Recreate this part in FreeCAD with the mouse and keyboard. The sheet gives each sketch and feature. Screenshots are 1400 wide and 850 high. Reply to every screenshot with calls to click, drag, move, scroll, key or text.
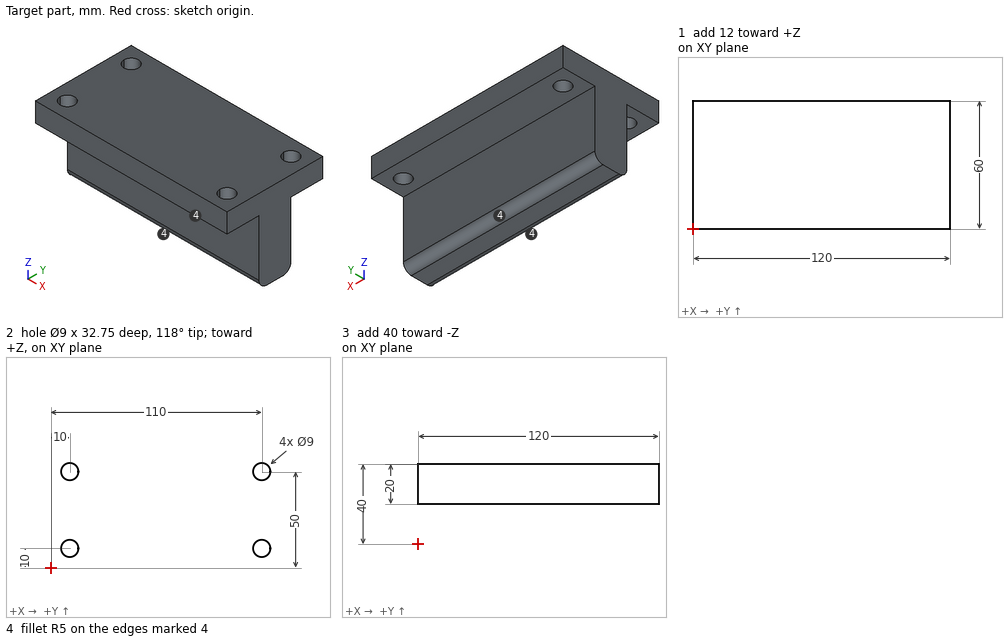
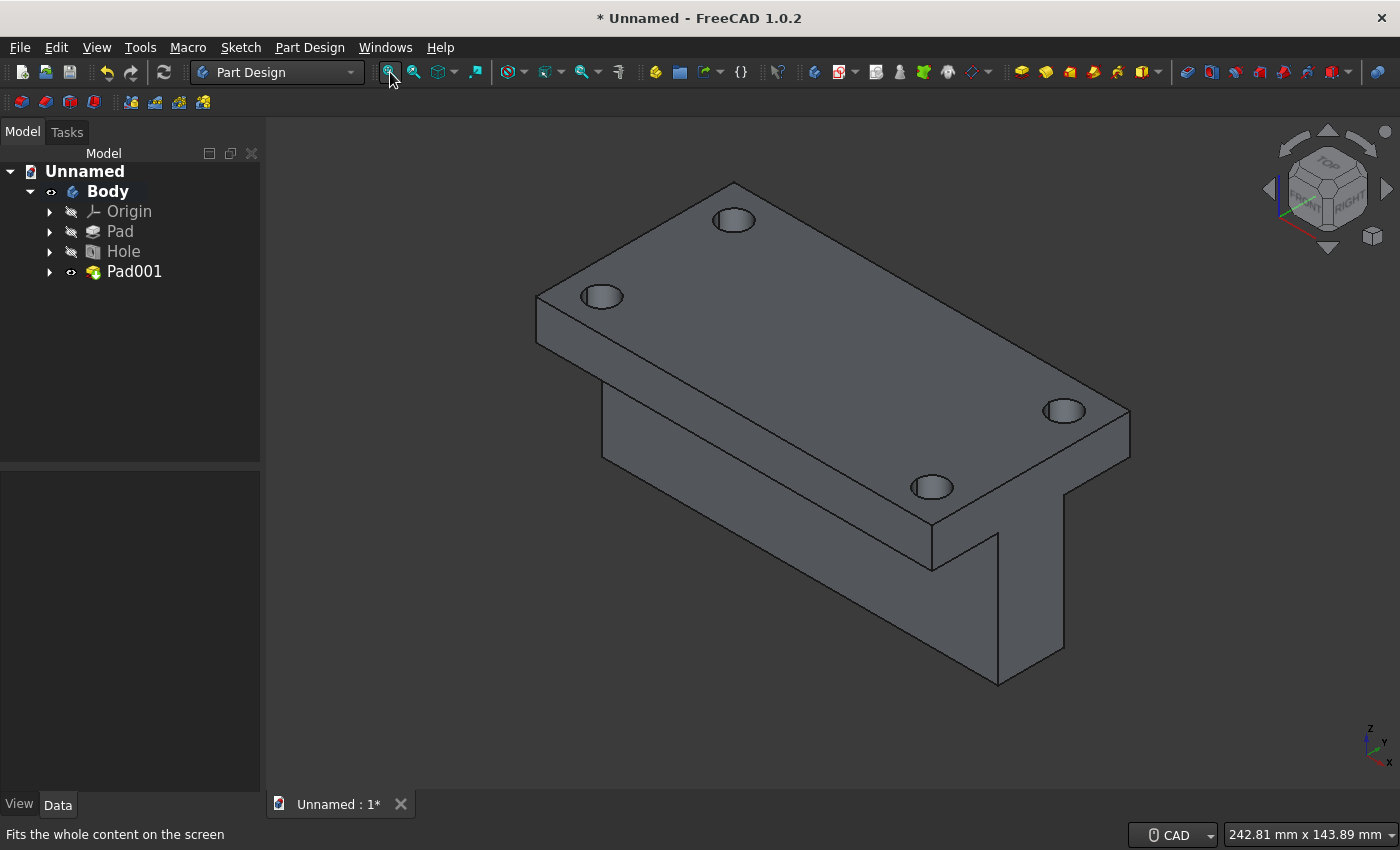
key(2)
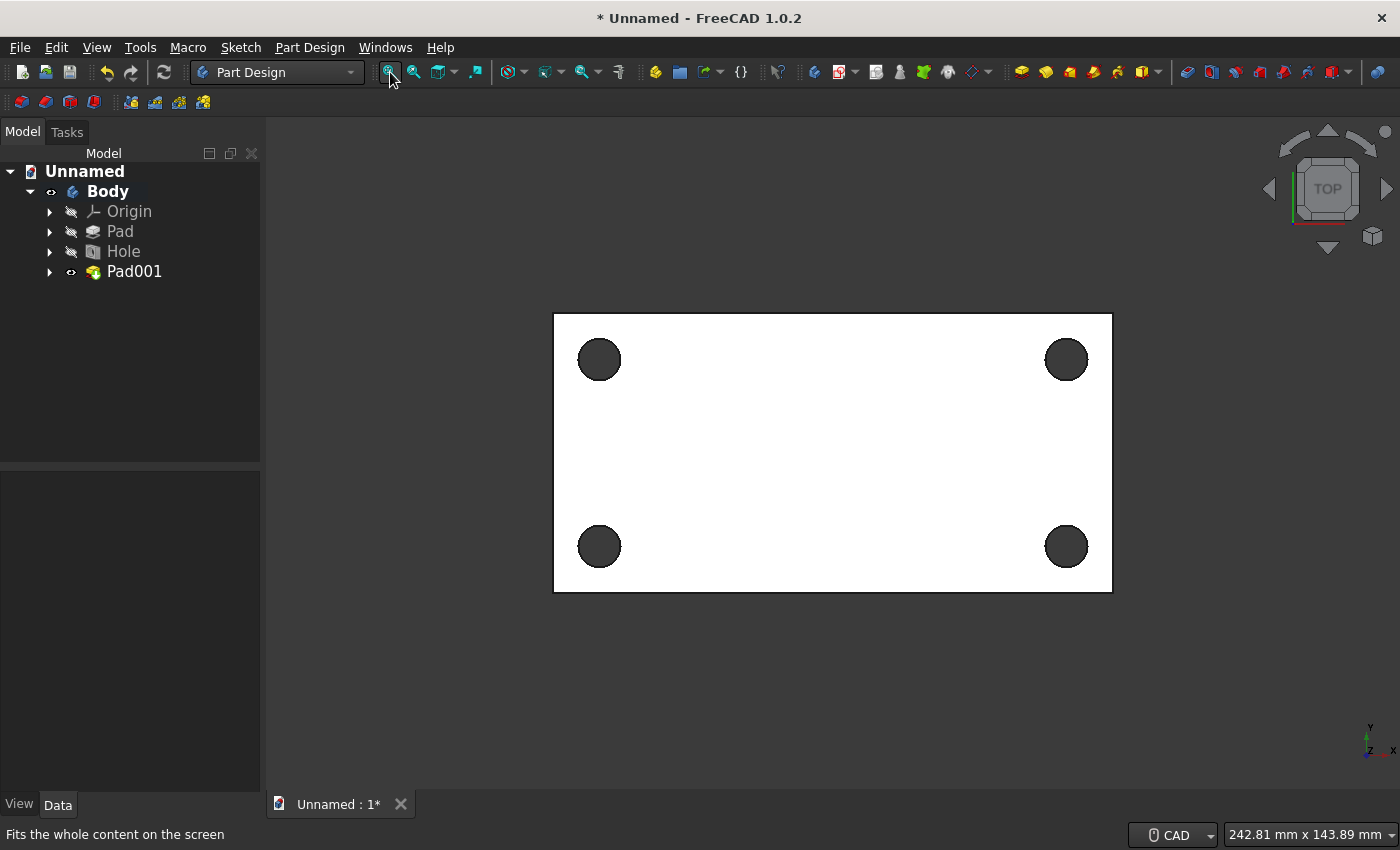
key(1)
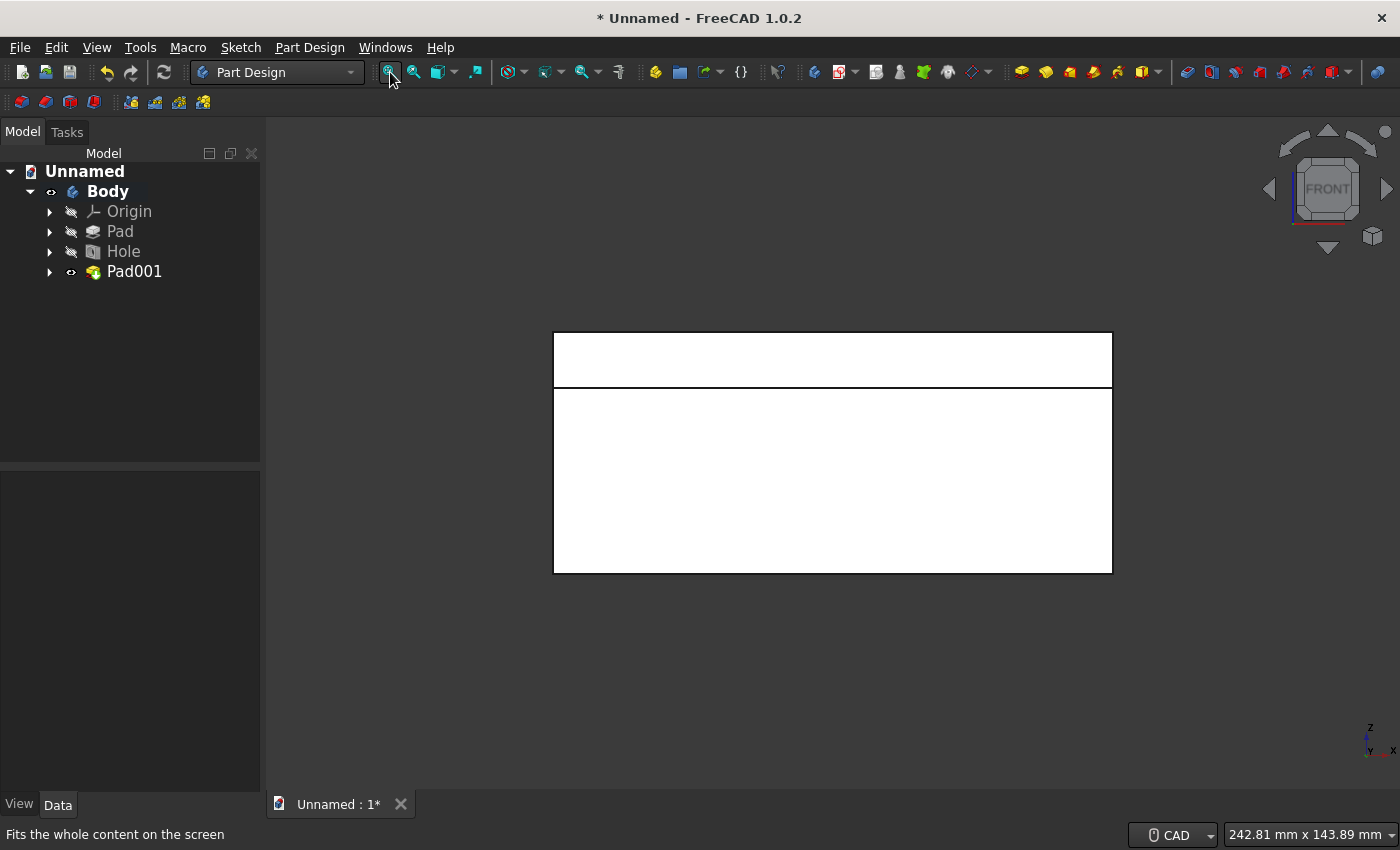
click(833, 573)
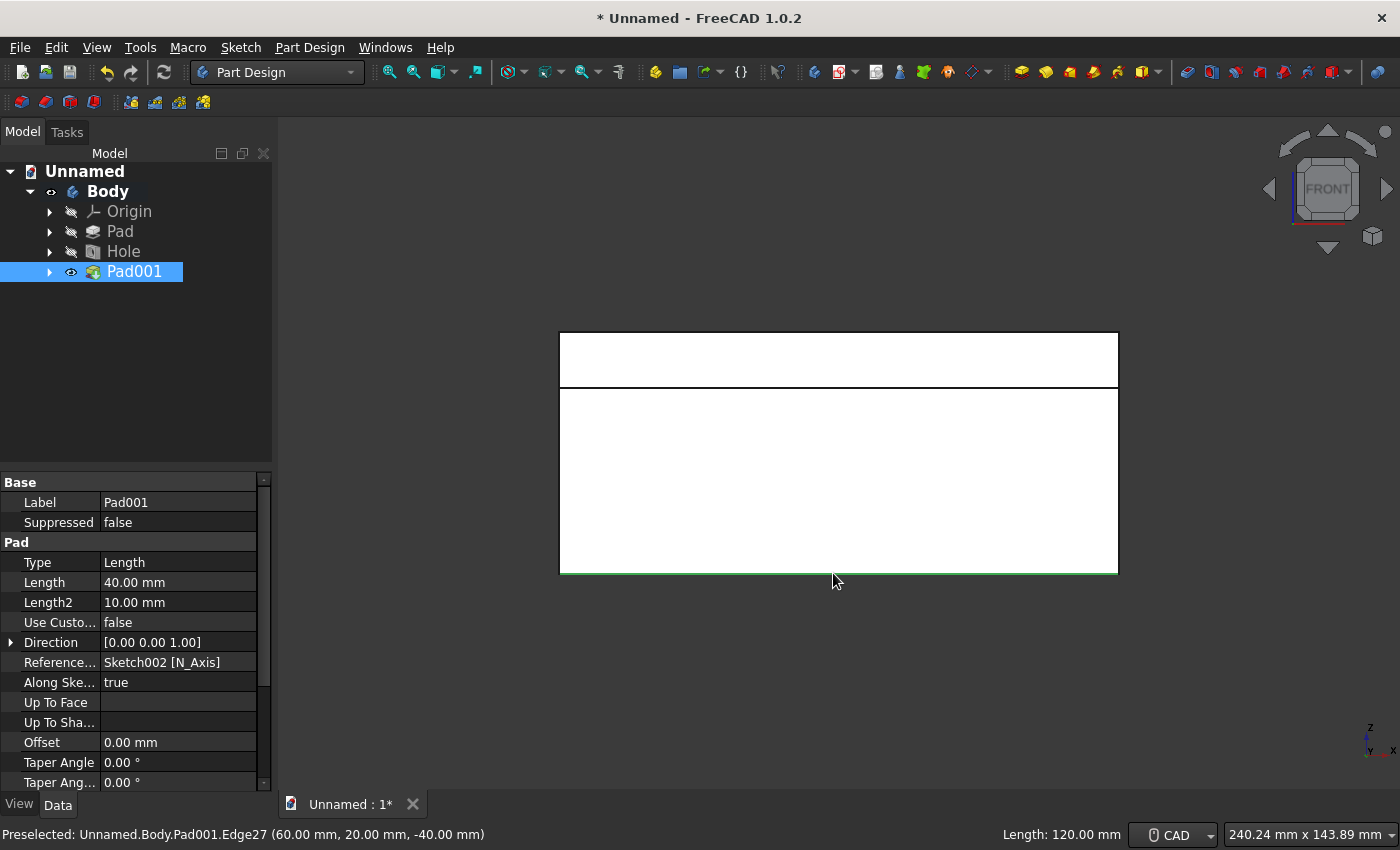
key(3)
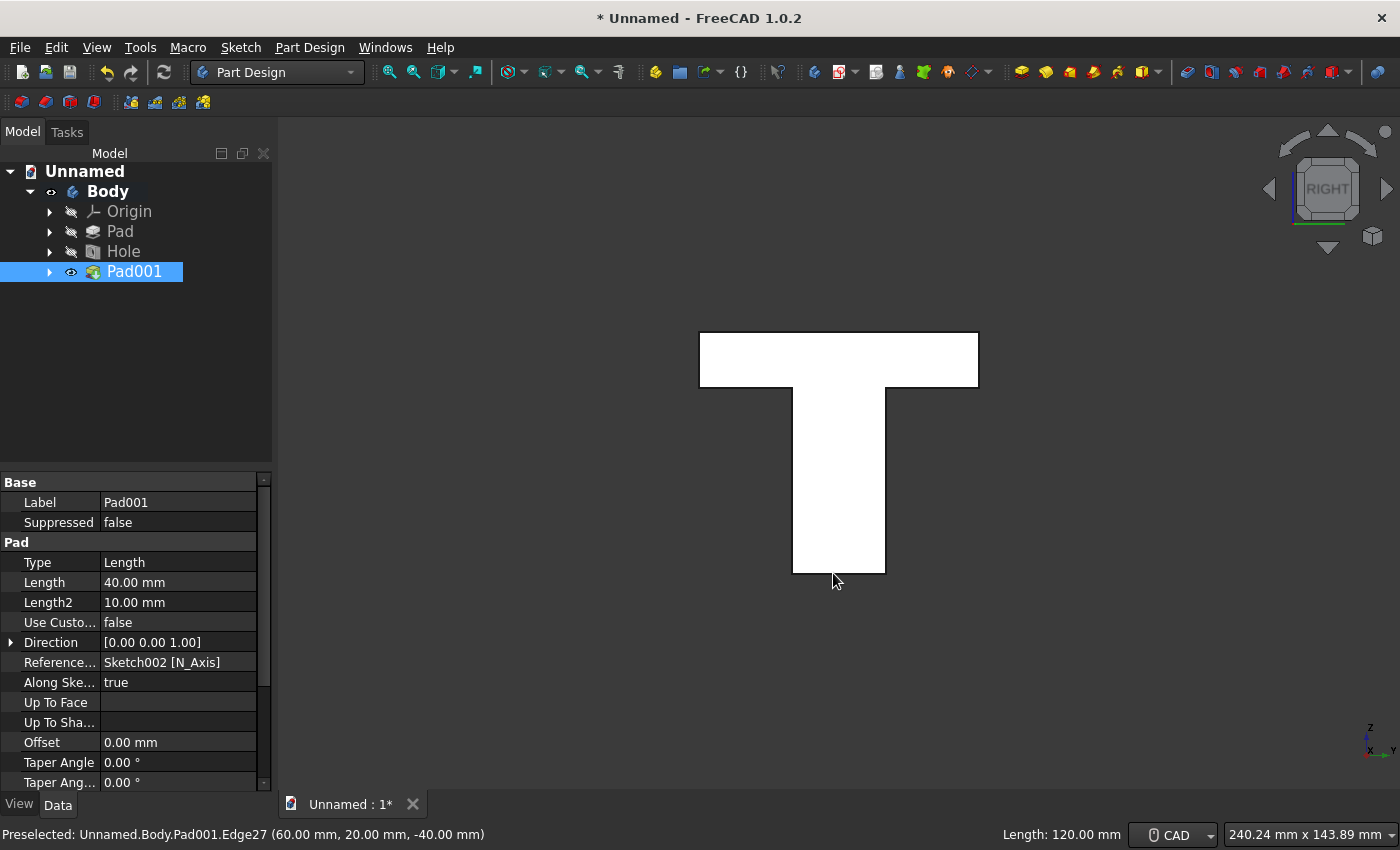
click(390, 72)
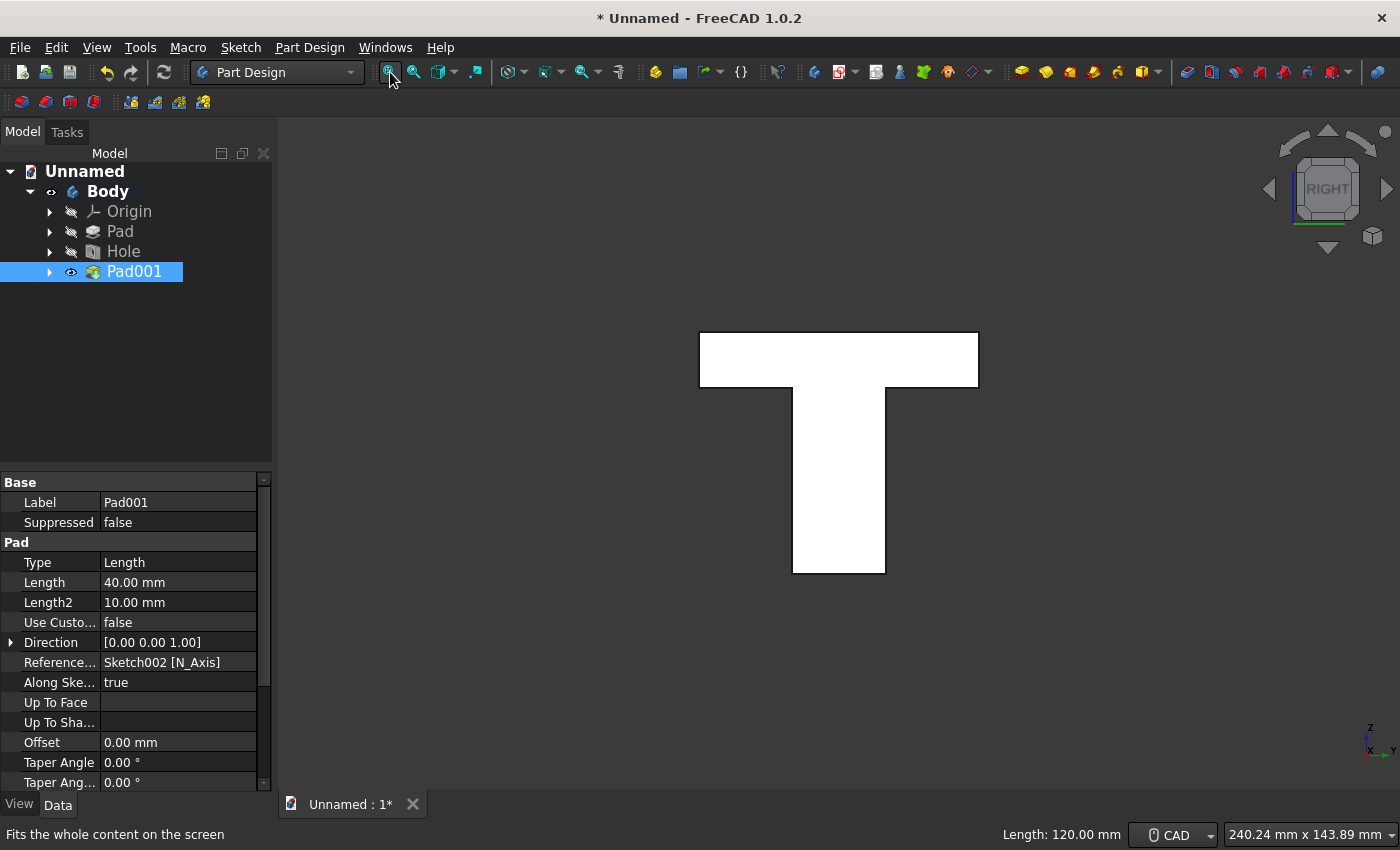
key(5)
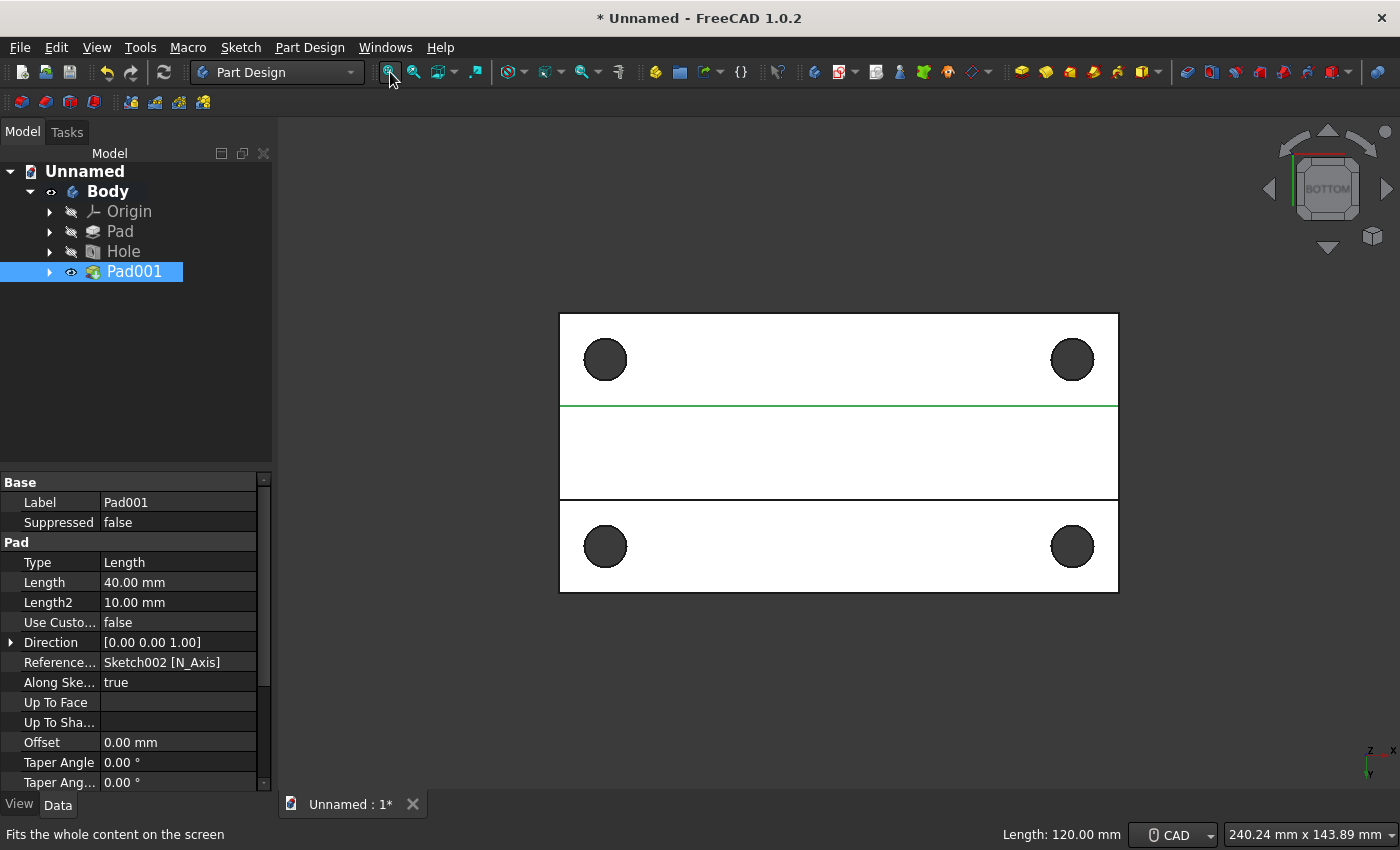
click(839, 499, ctrl)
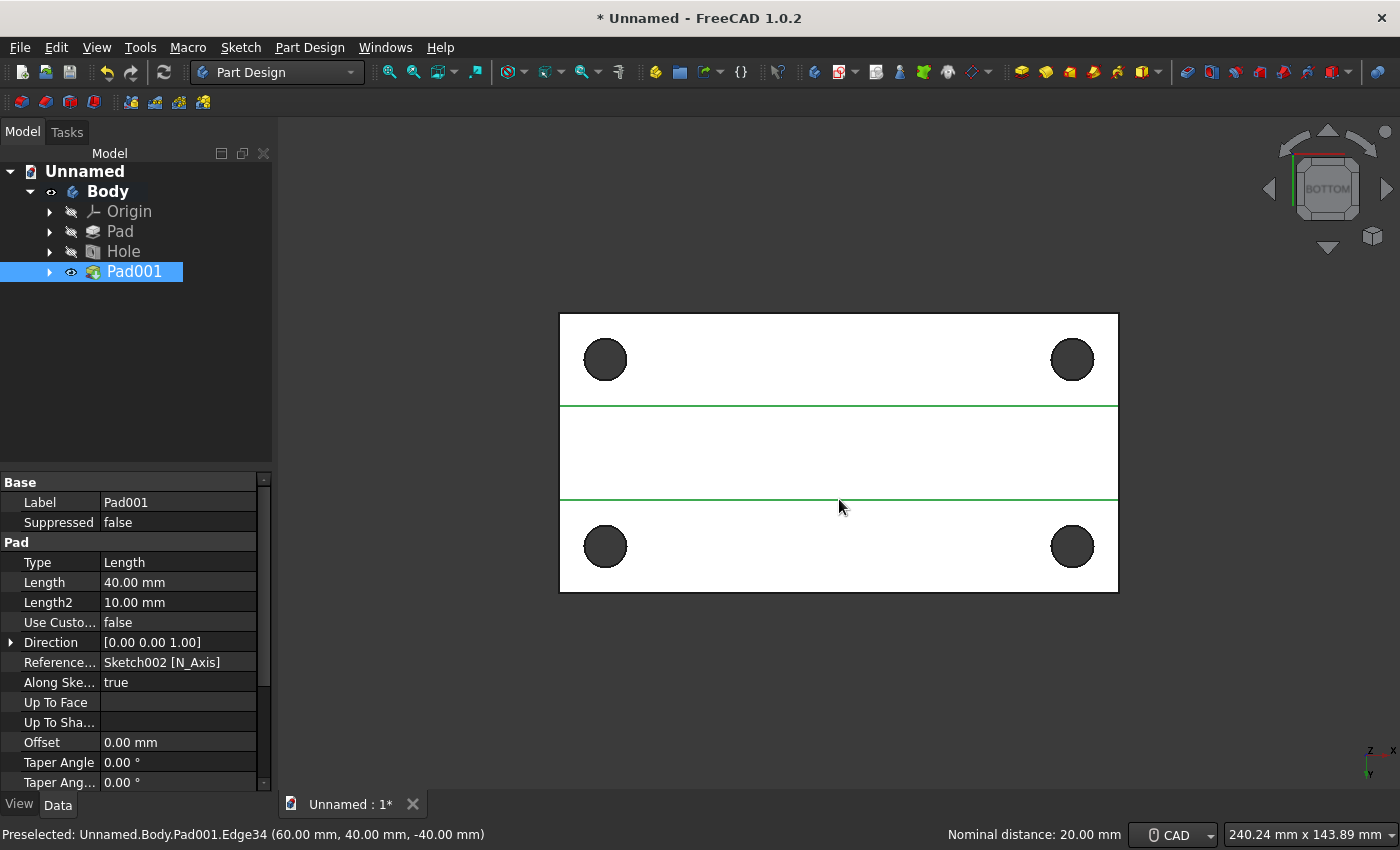
click(22, 102)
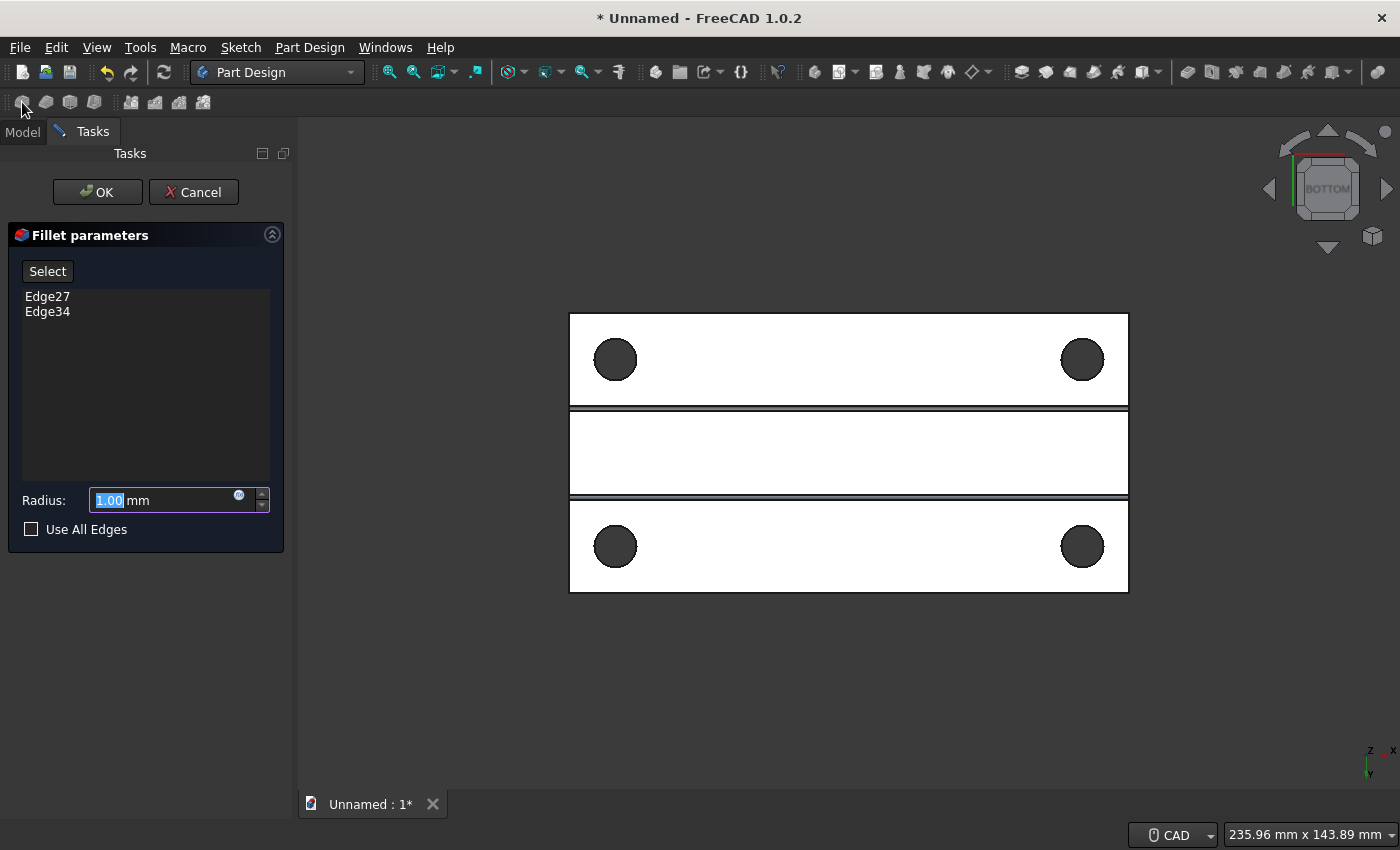
text(5)
key(Tab)